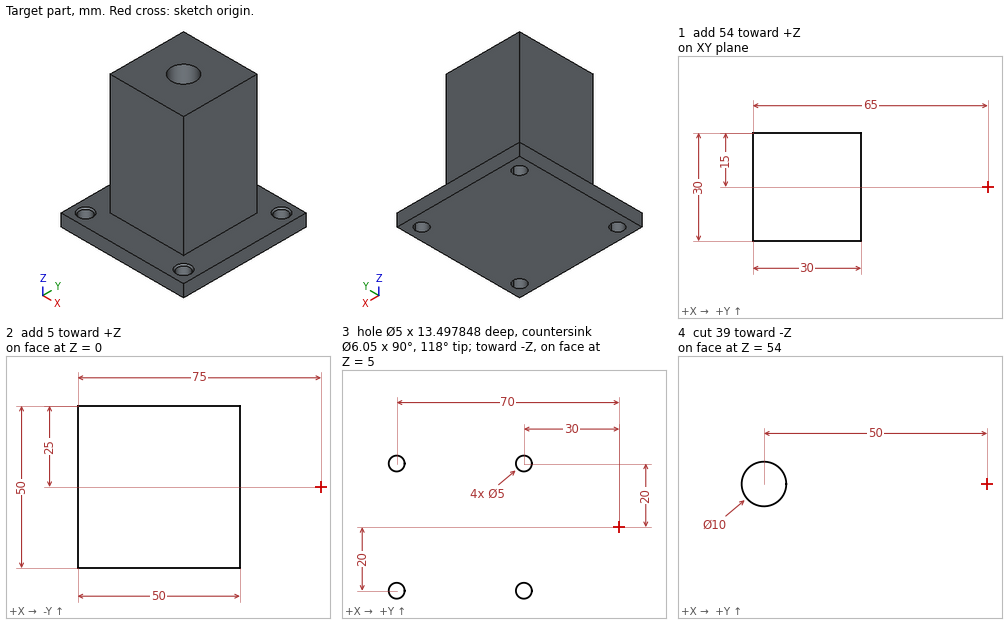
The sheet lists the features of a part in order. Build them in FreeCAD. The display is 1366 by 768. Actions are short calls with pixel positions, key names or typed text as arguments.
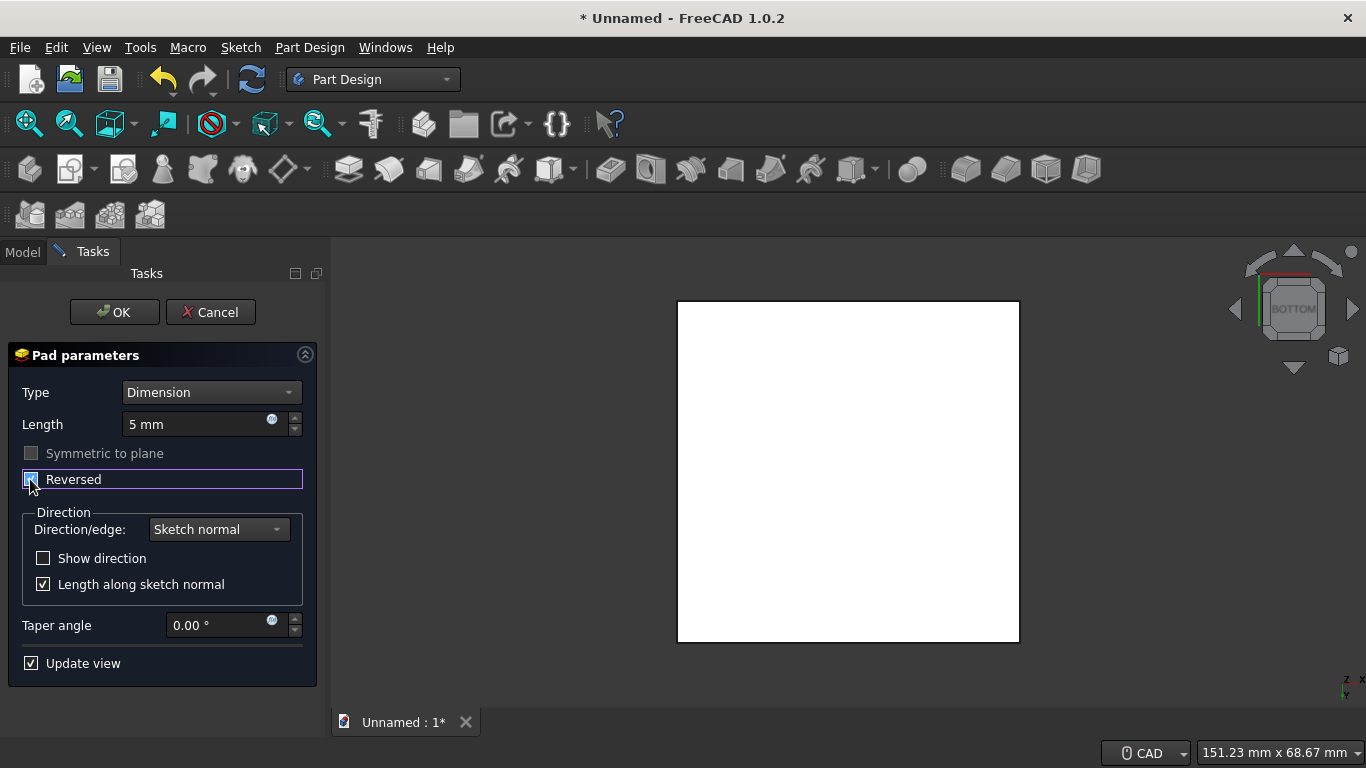
click(115, 312)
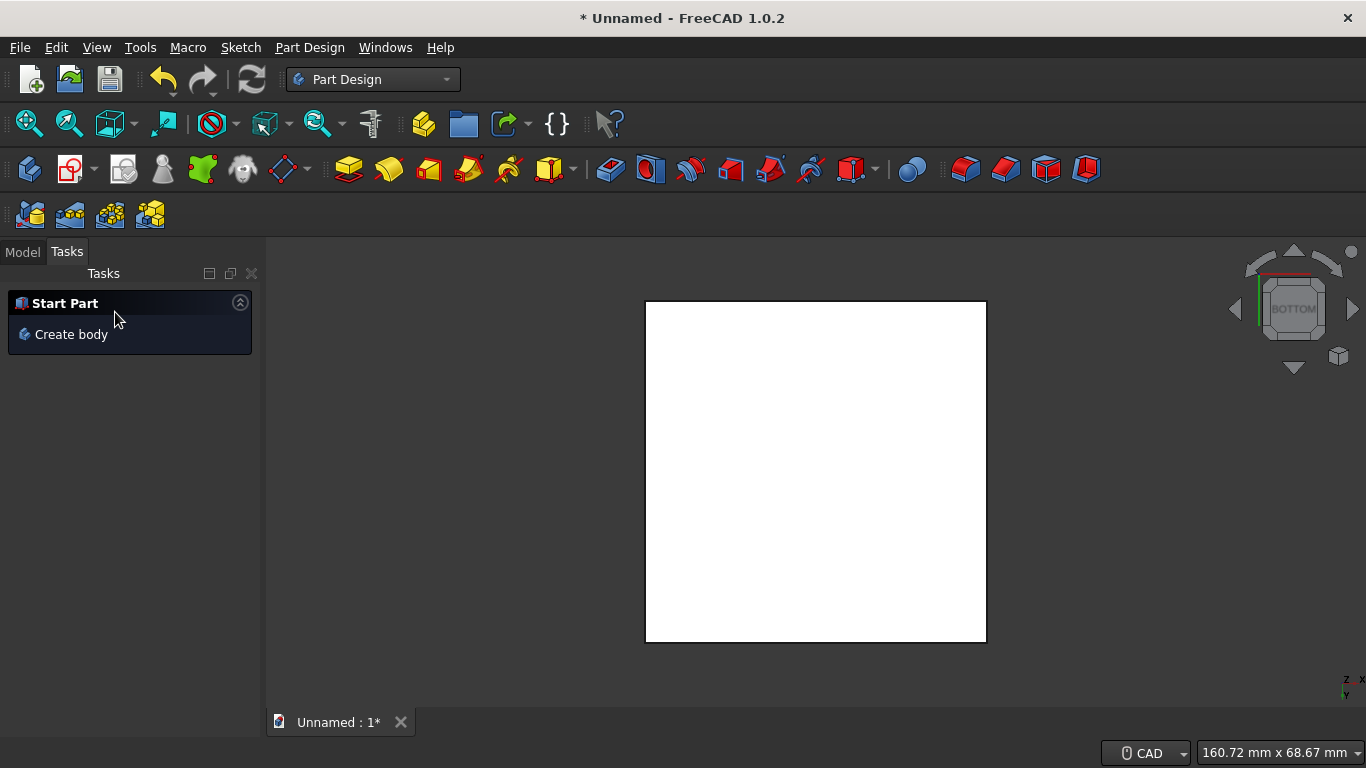
key(0)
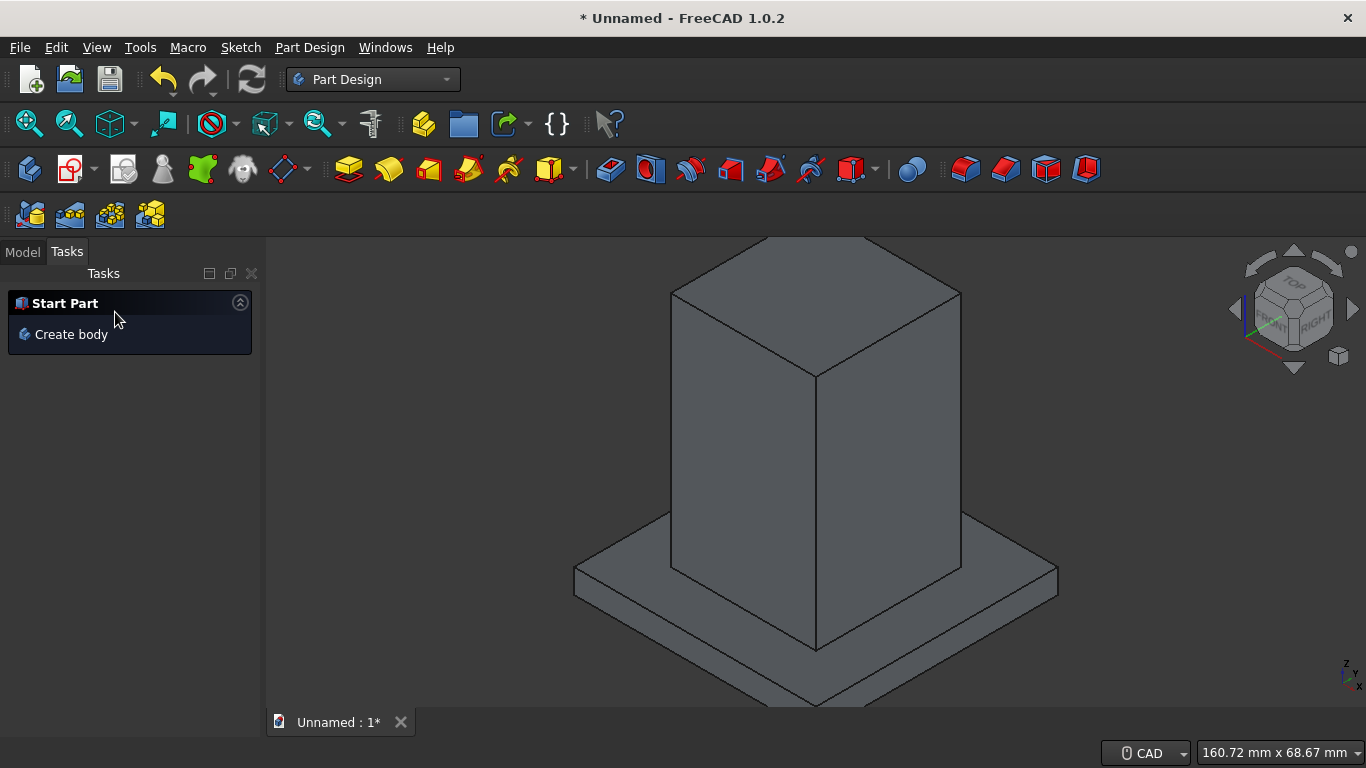
key(v)
key(f)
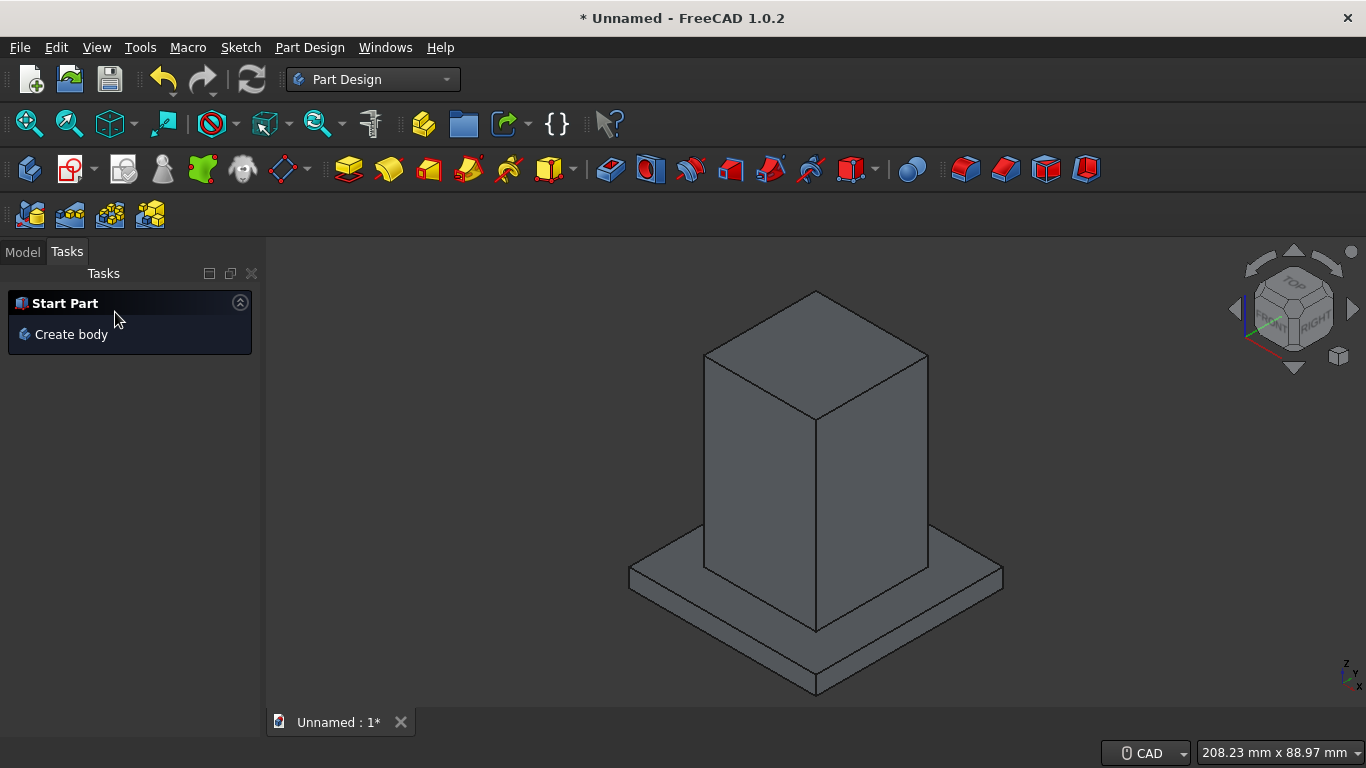
click(789, 643)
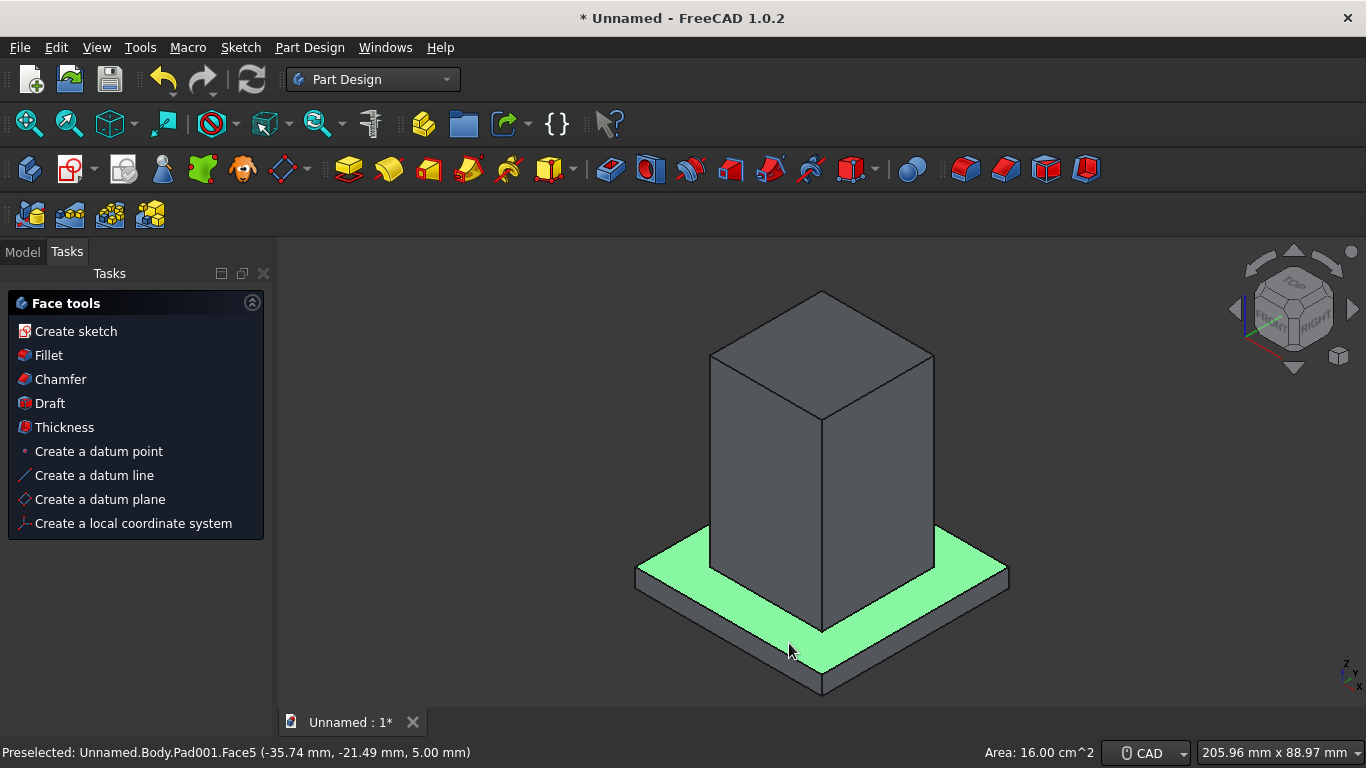
click(70, 170)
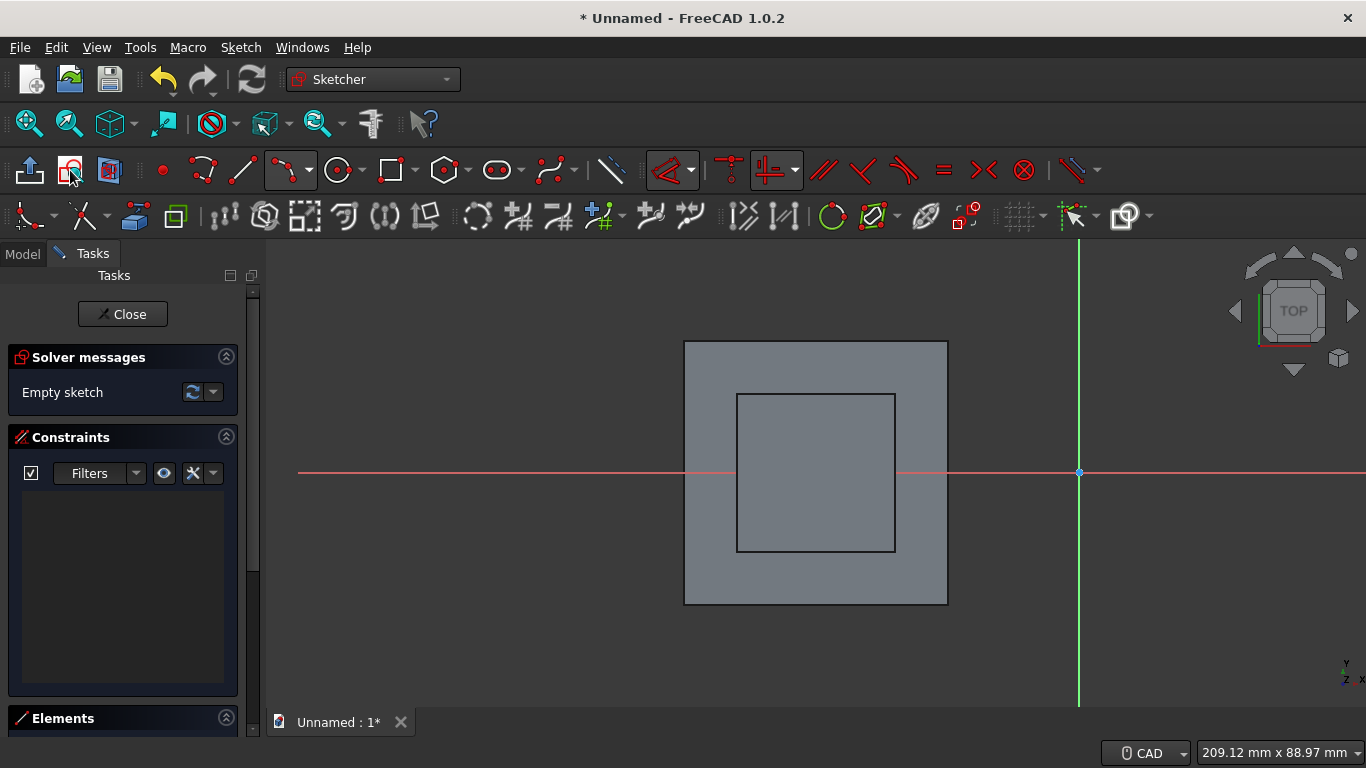
key(q)
key(s)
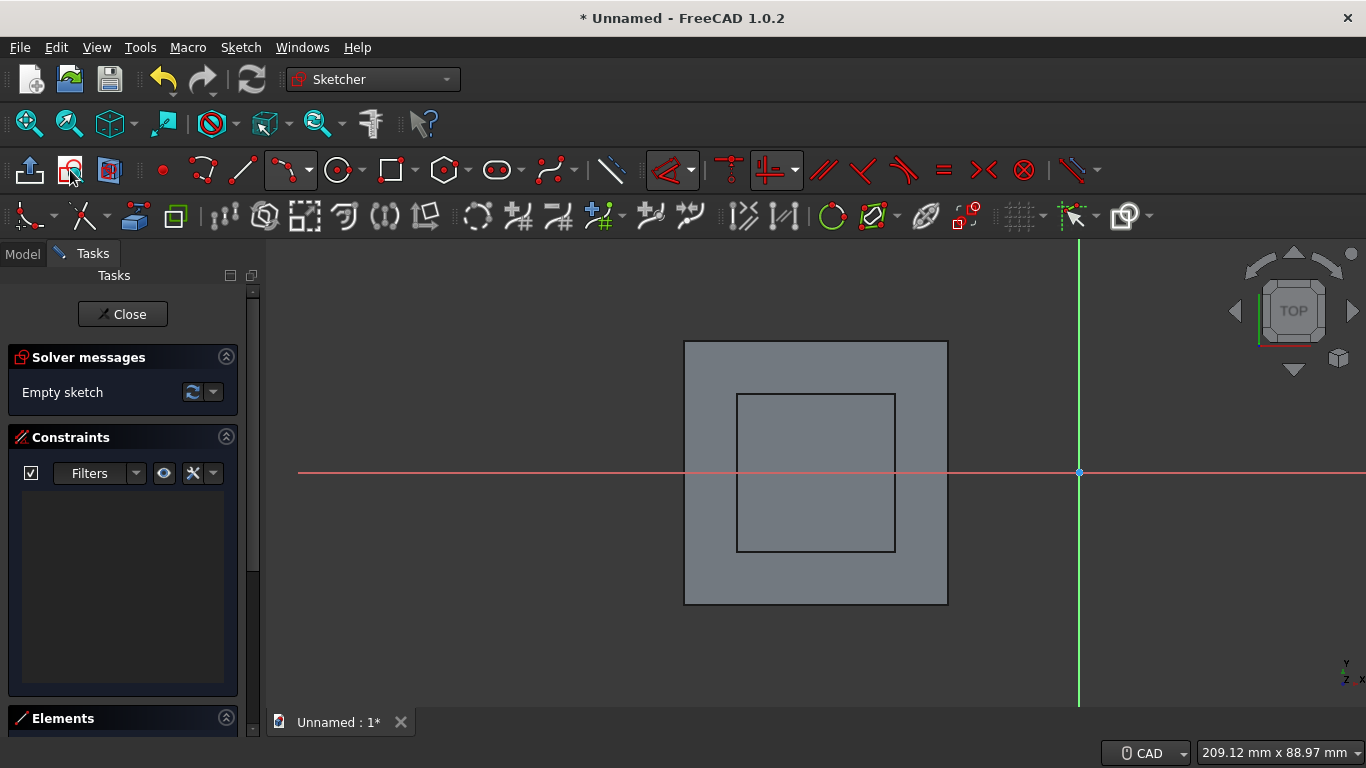
key(g)
key(c)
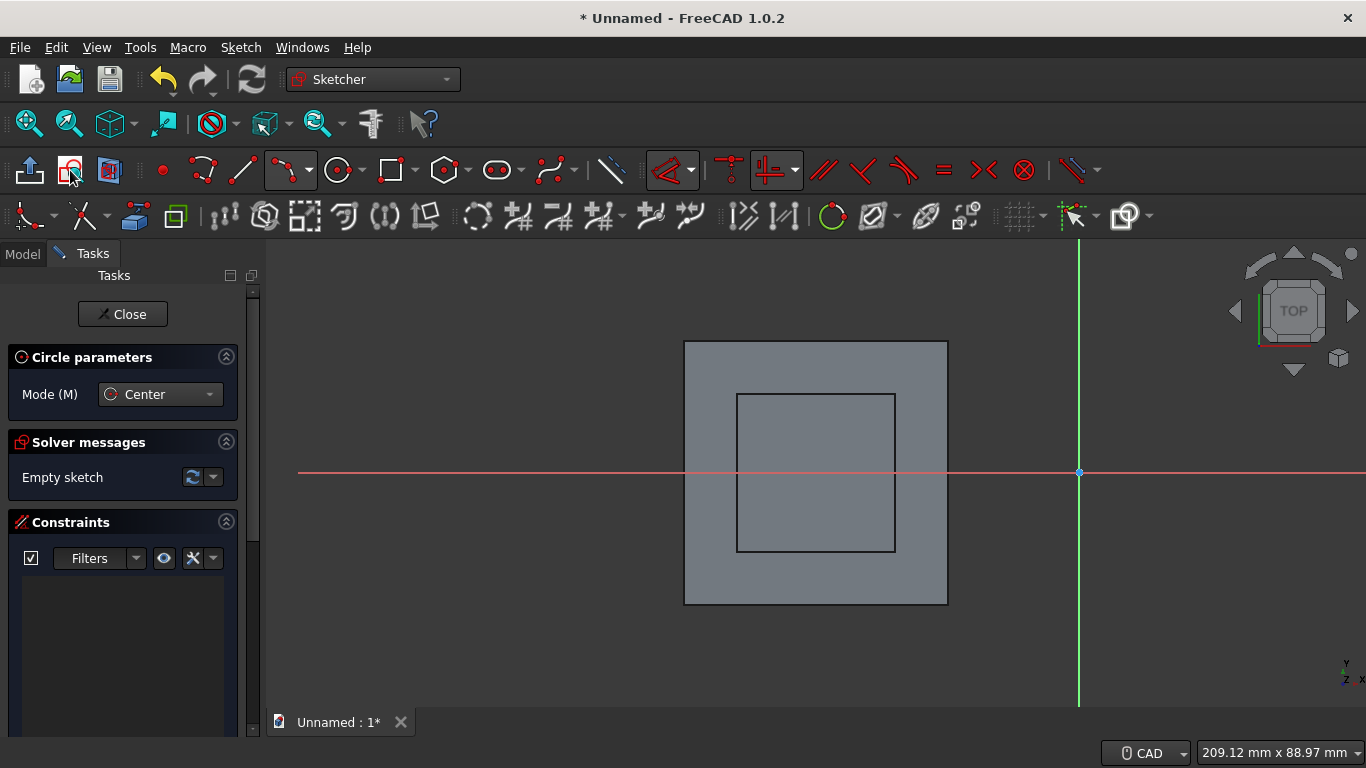
scroll(921, 368, up, 3)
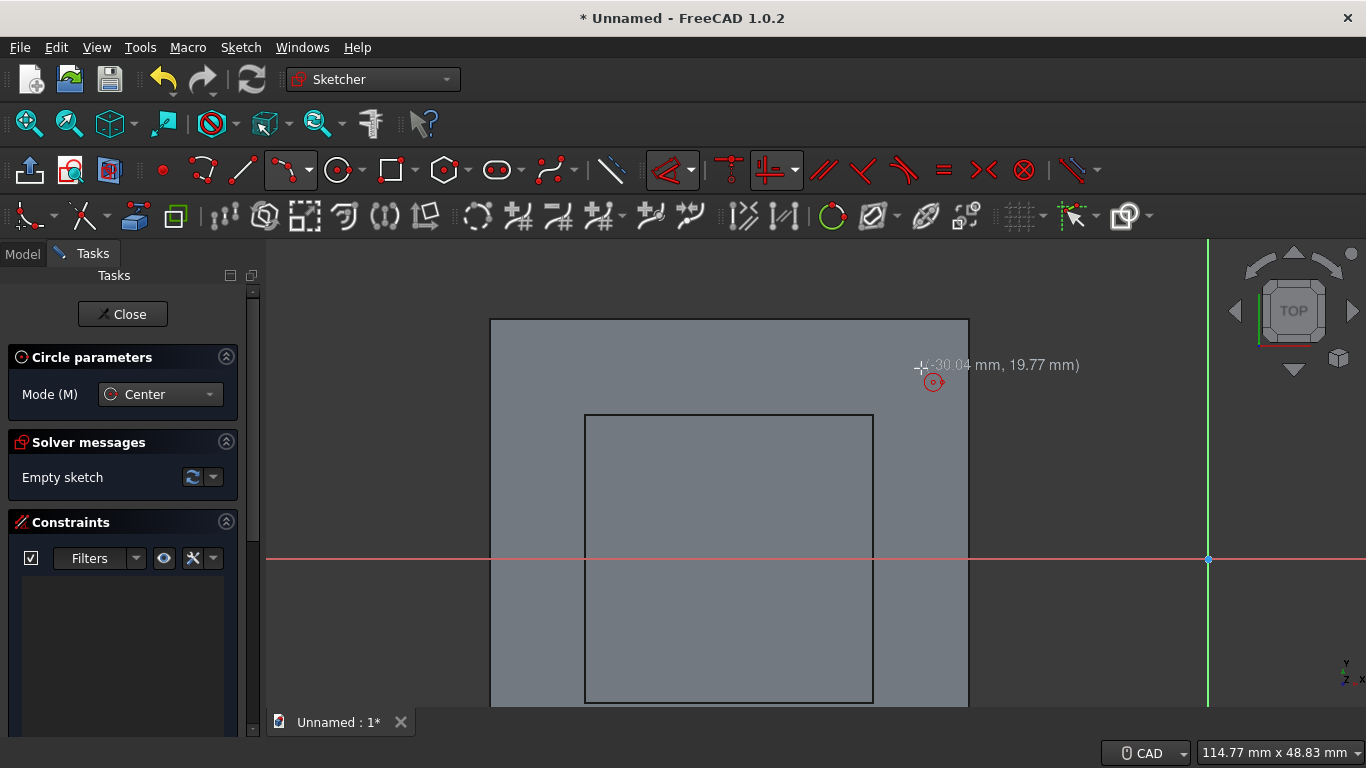
click(921, 367)
click(938, 350)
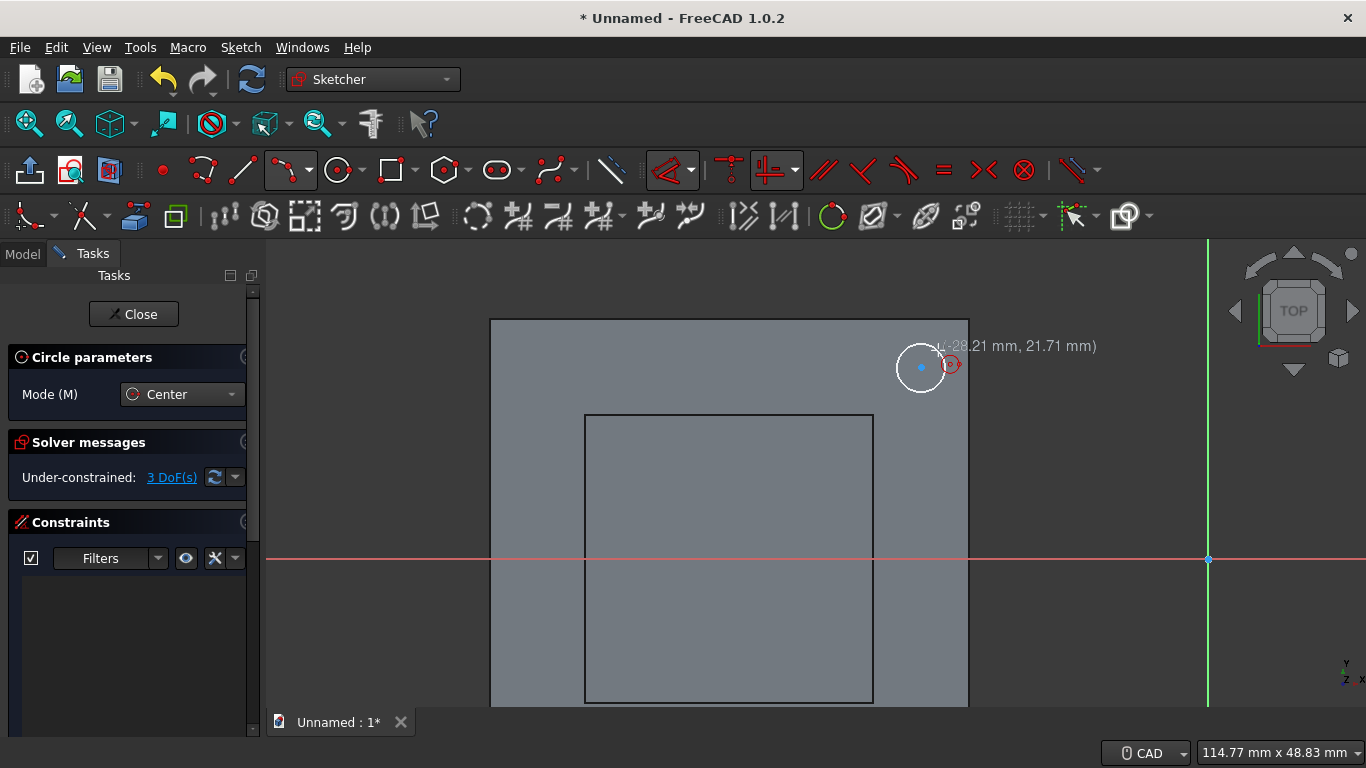
click(537, 367)
click(554, 350)